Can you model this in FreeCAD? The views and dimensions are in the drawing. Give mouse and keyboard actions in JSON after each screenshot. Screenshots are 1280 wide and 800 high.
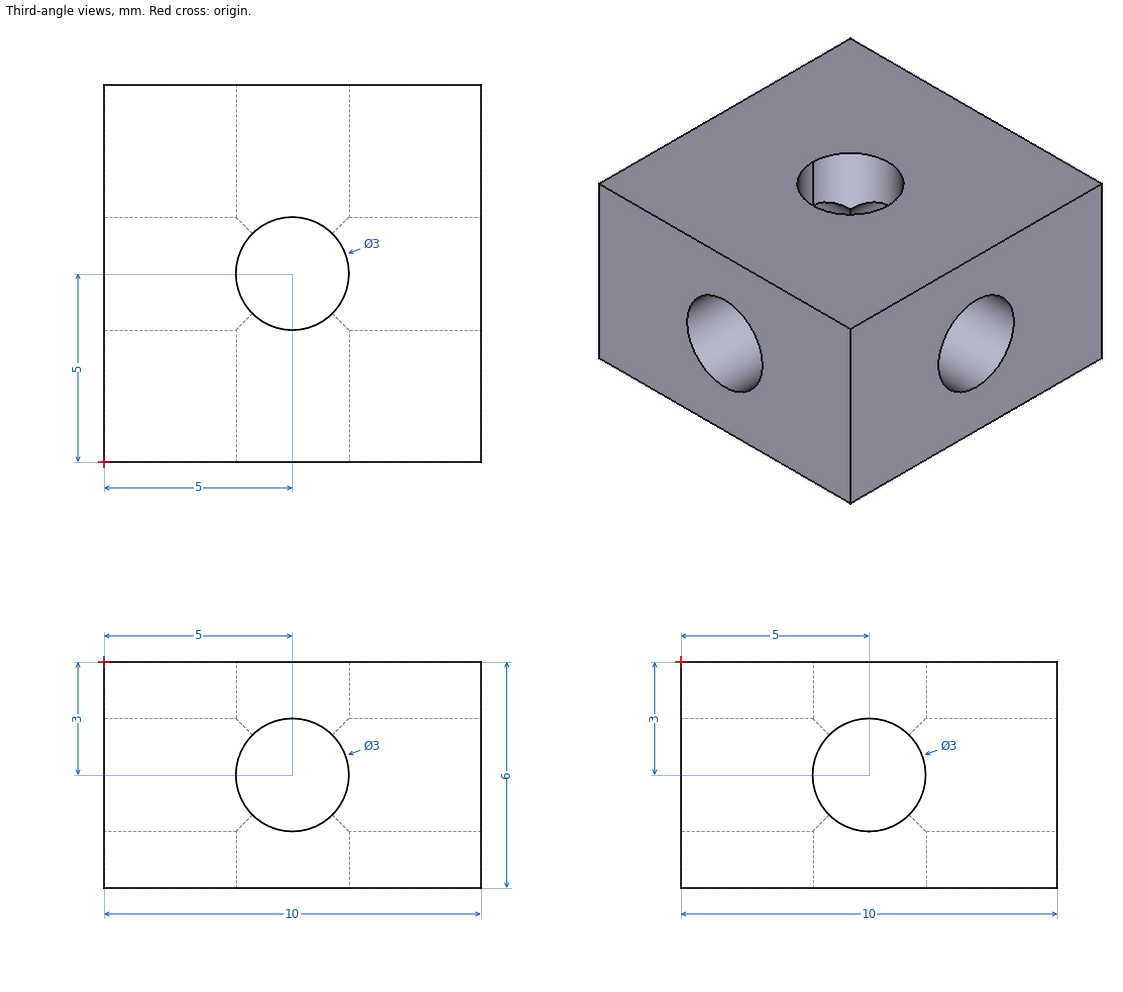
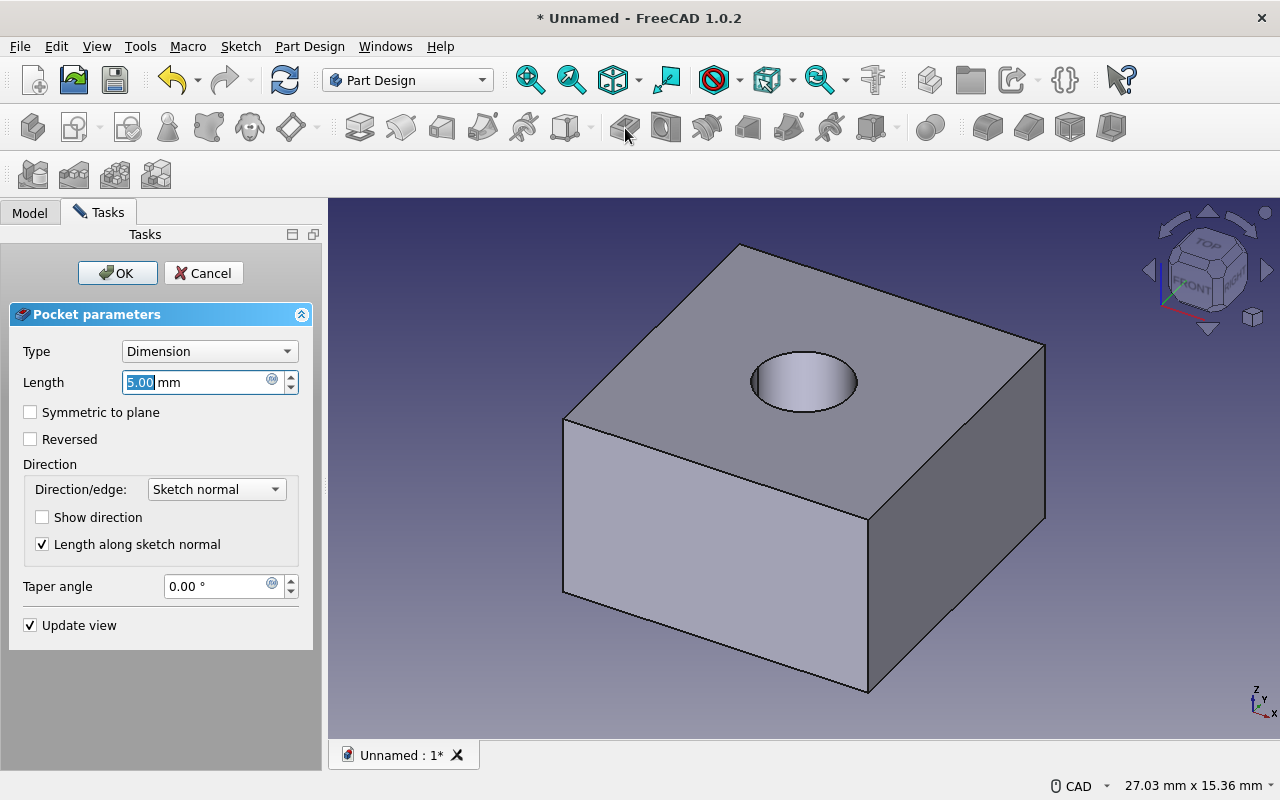
{"action": "left_click", "coordinate": [210, 352]}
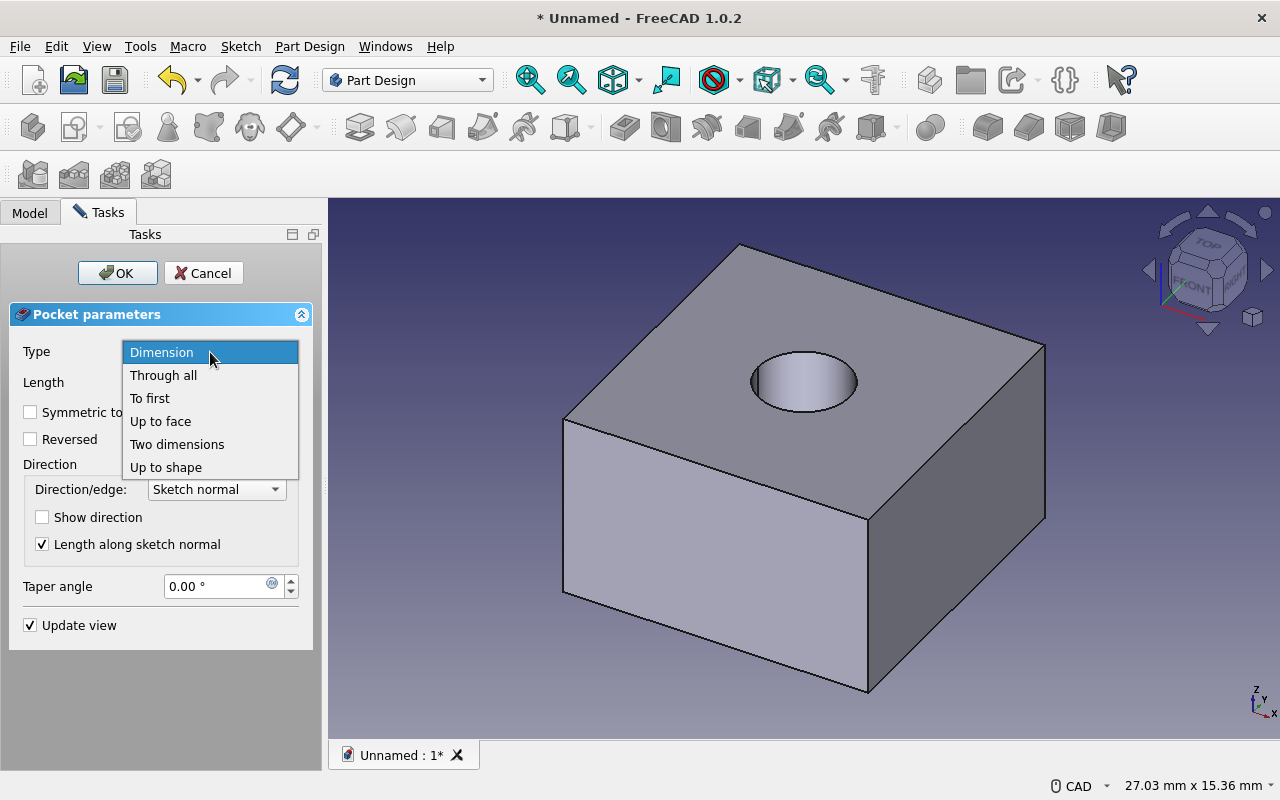
{"action": "left_click", "coordinate": [208, 376]}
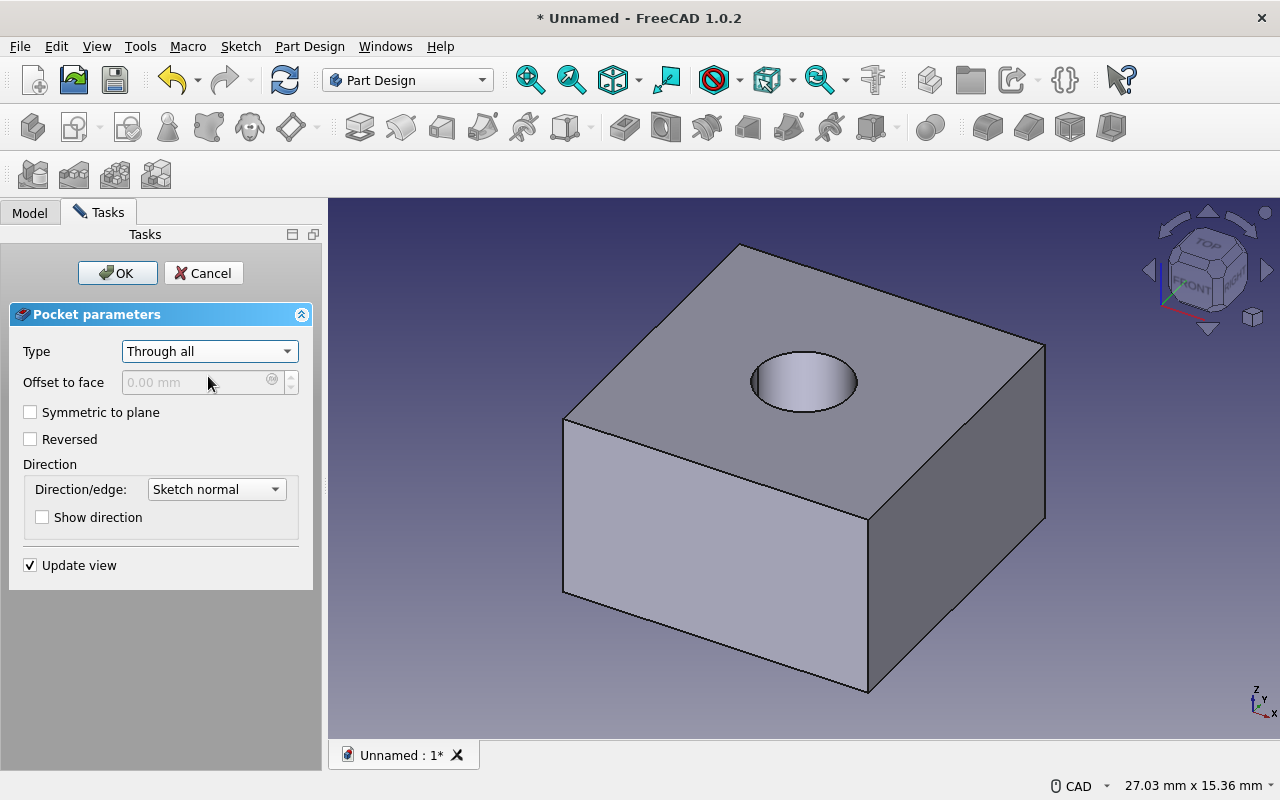
{"action": "left_click", "coordinate": [118, 273]}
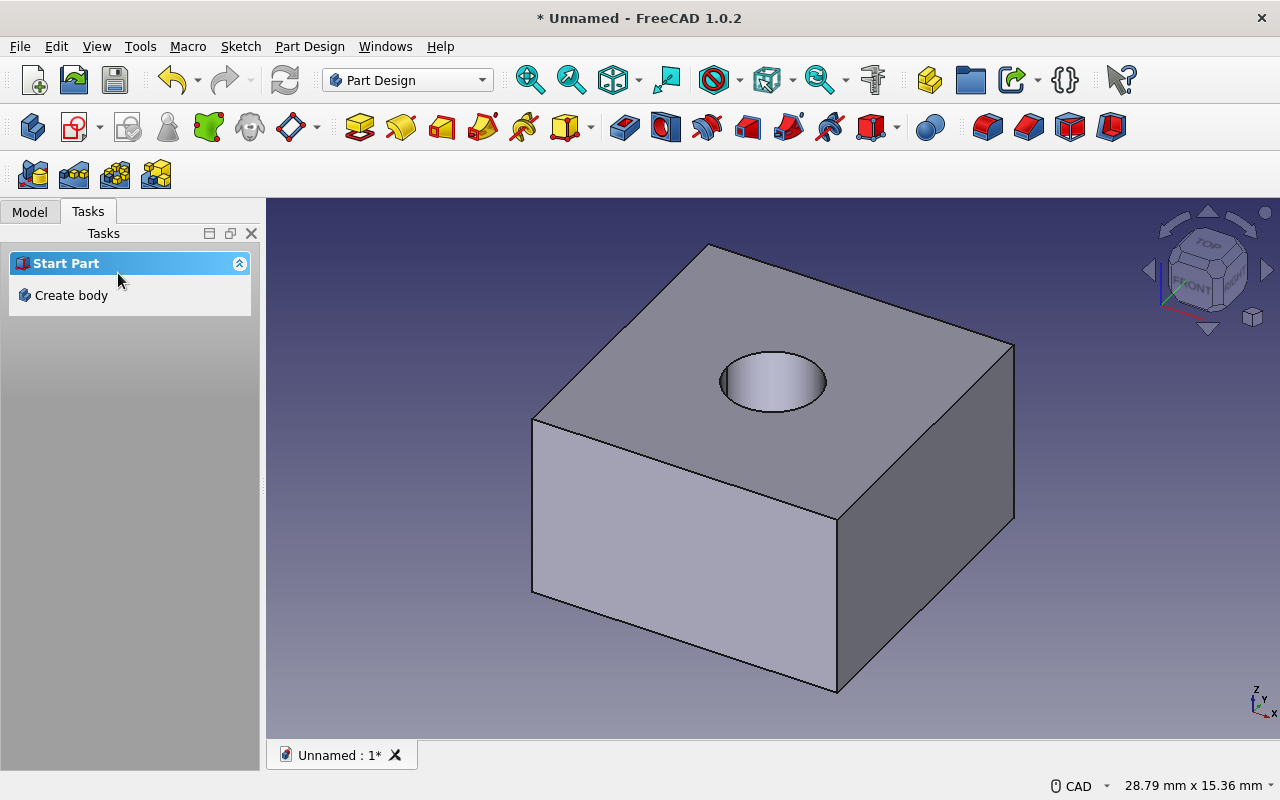
{"action": "key", "text": "4"}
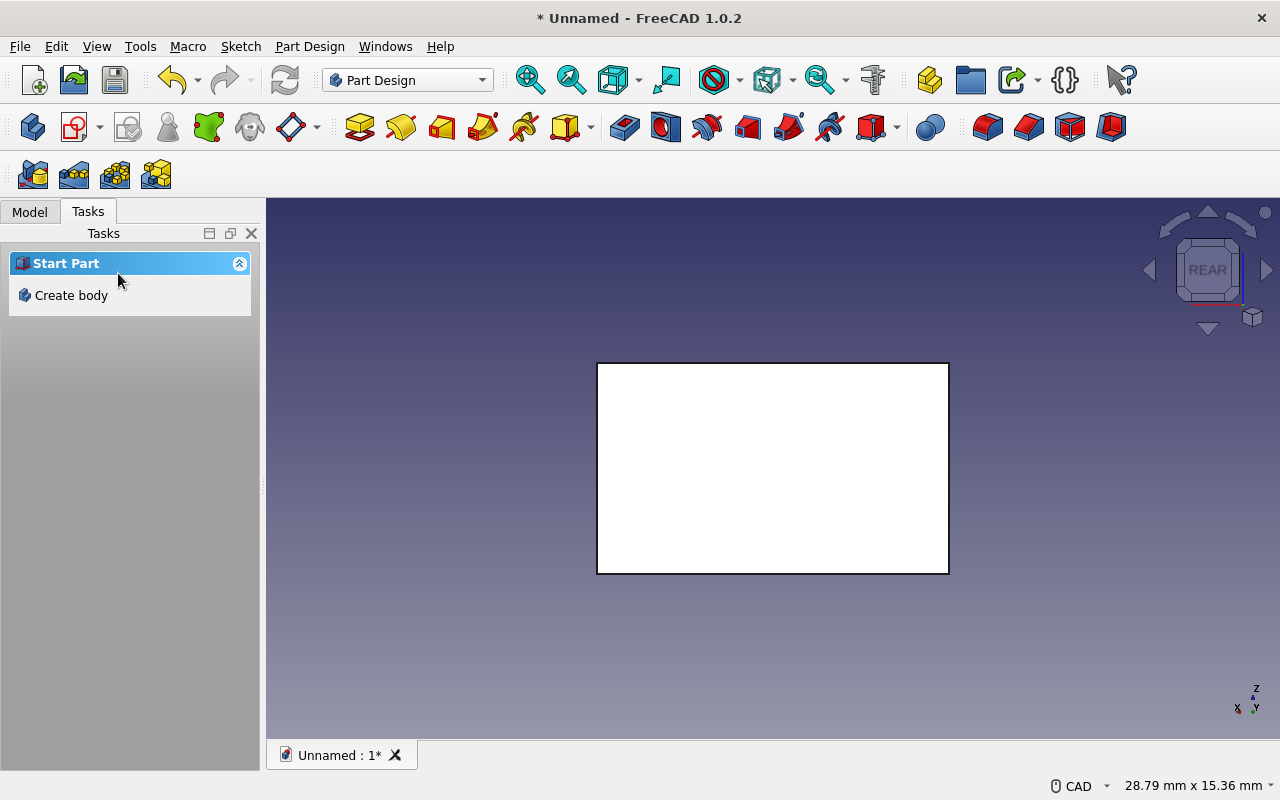
{"action": "left_click", "coordinate": [531, 80]}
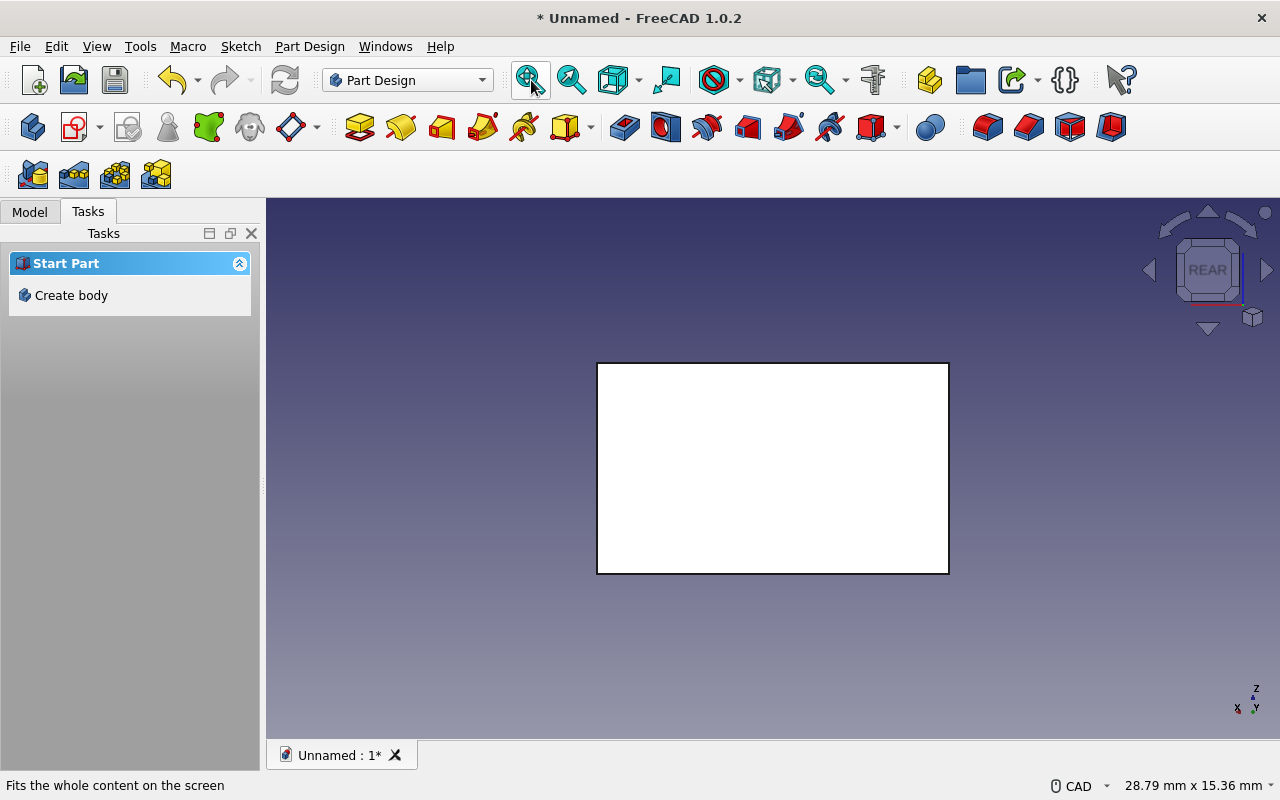
{"action": "left_click", "coordinate": [723, 468]}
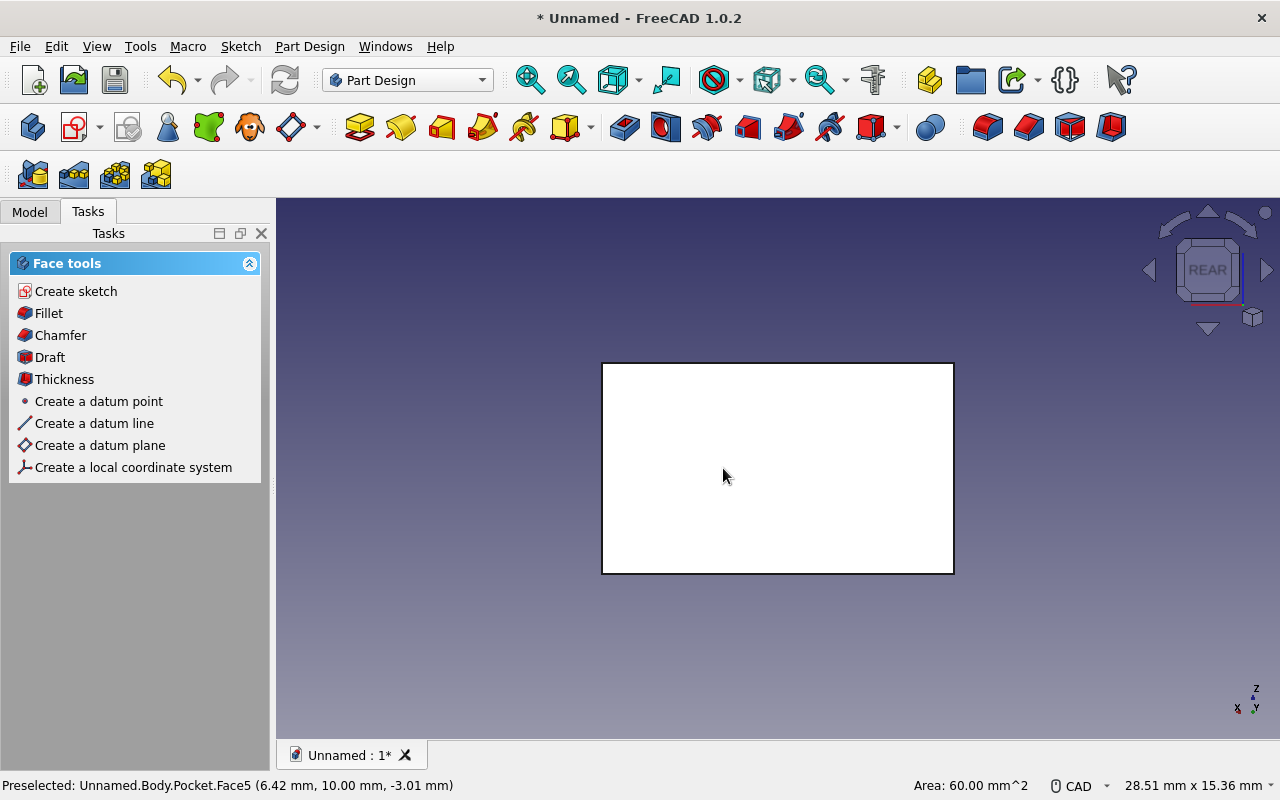
{"action": "left_click", "coordinate": [74, 128]}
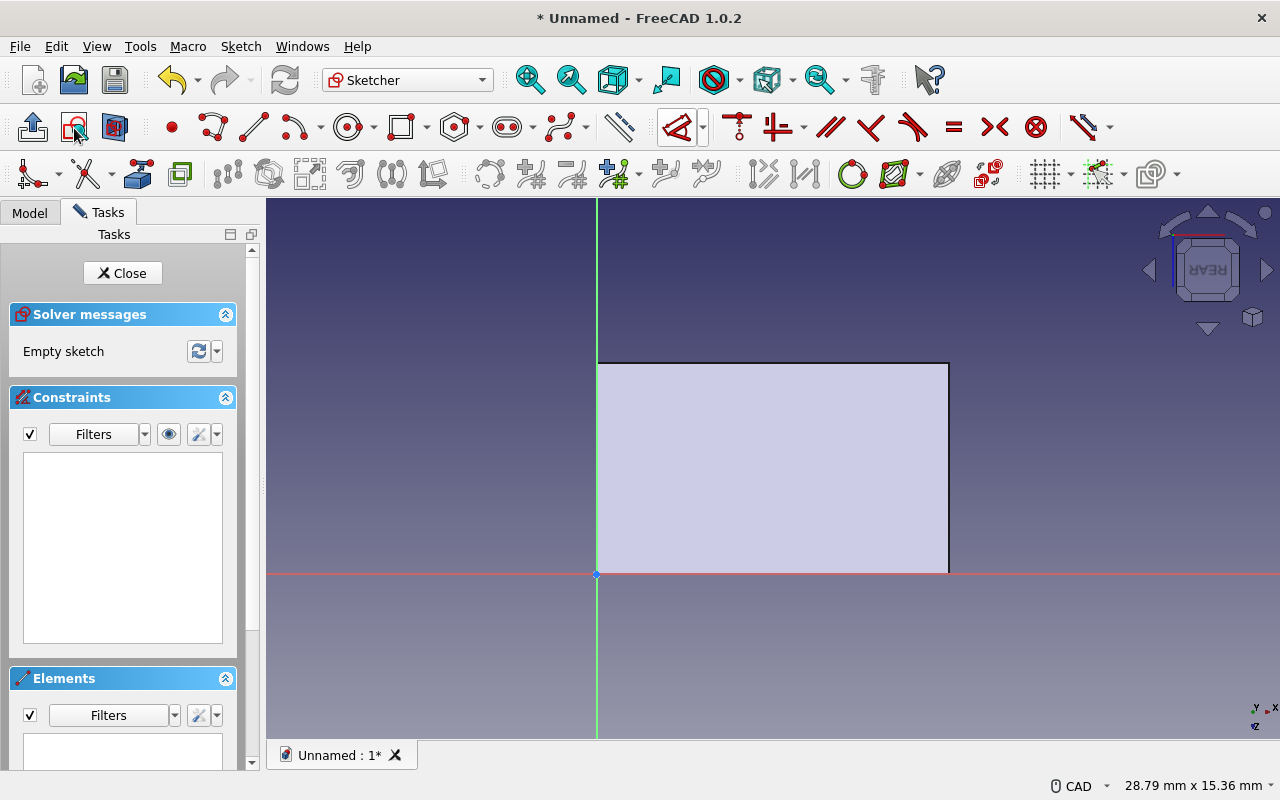
{"action": "scroll", "coordinate": [717, 516], "scroll_direction": "up", "scroll_amount": 4}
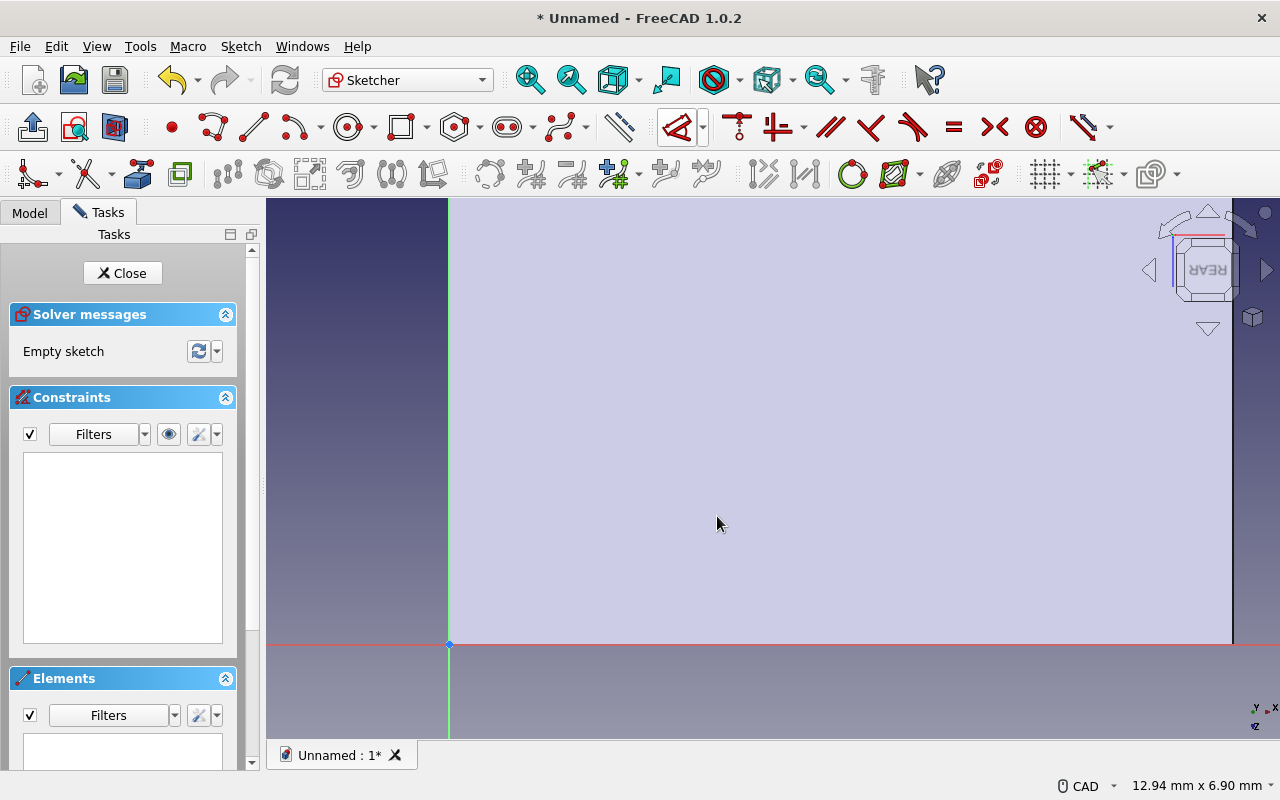
{"action": "left_click", "coordinate": [348, 128]}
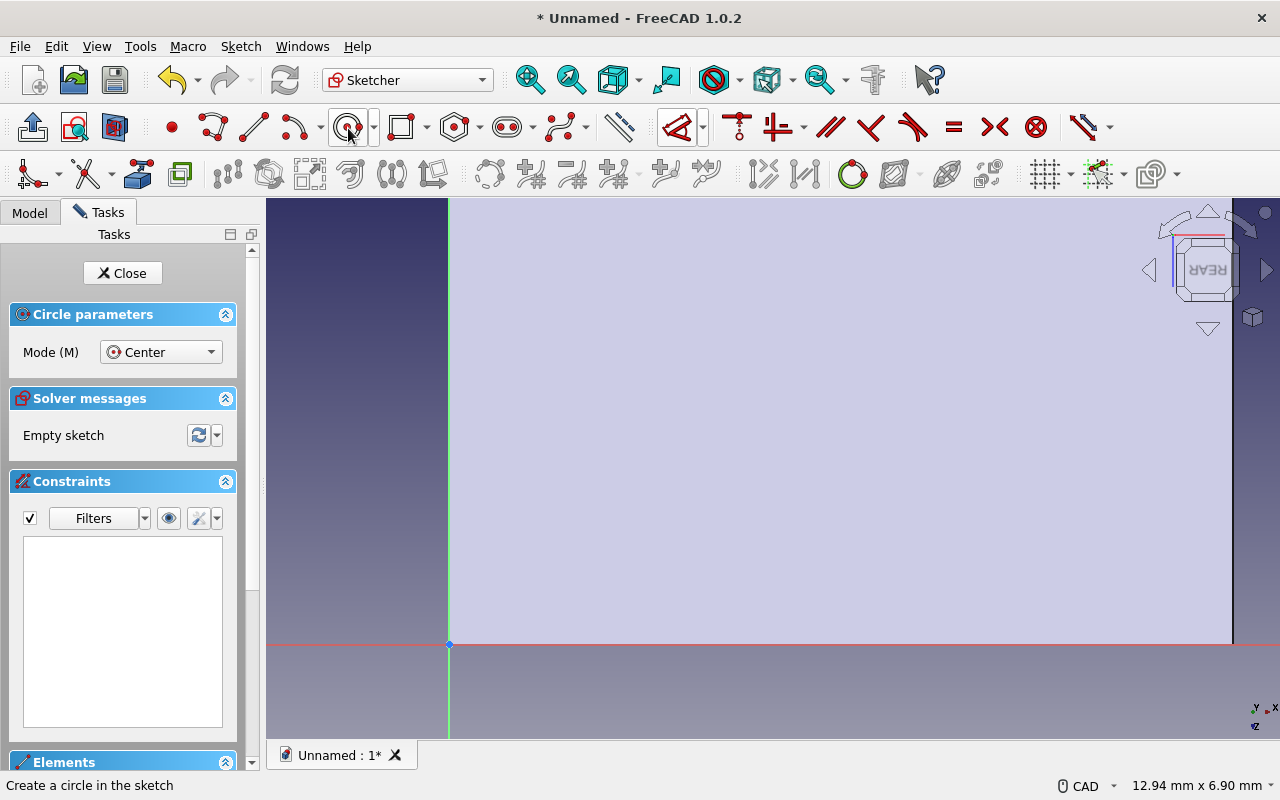
{"action": "left_click", "coordinate": [841, 410]}
{"action": "mouse_move", "coordinate": [924, 326]}